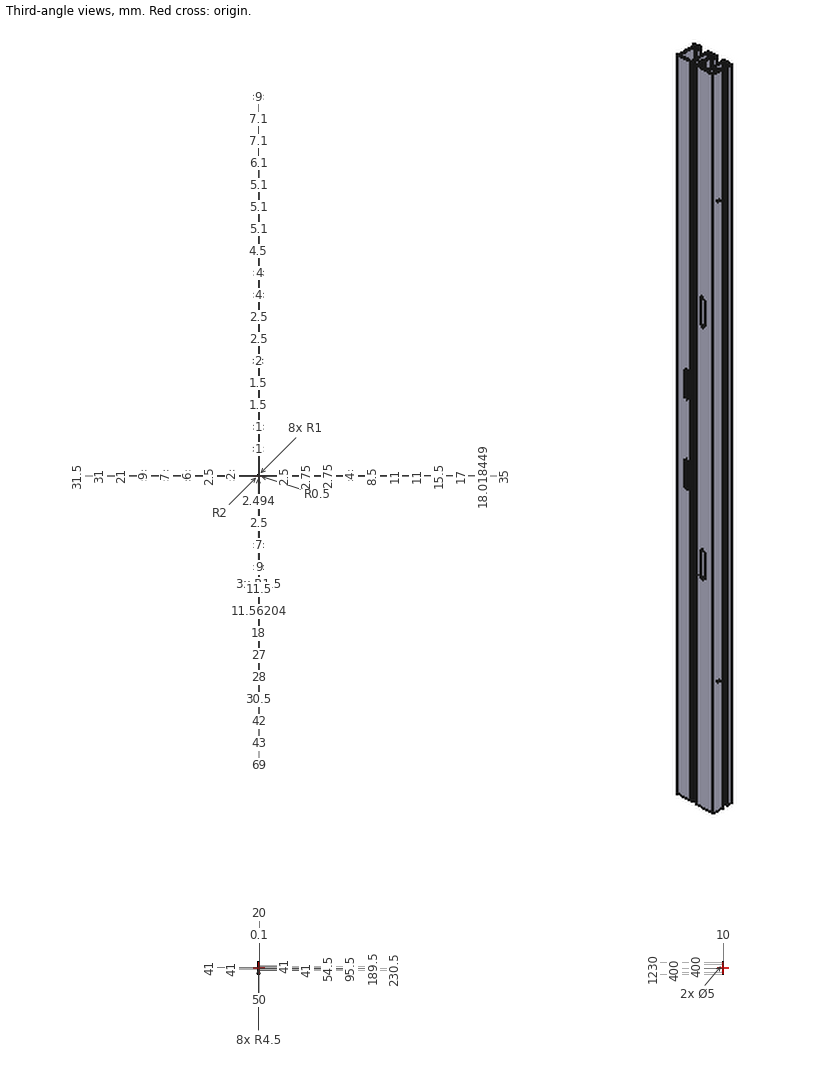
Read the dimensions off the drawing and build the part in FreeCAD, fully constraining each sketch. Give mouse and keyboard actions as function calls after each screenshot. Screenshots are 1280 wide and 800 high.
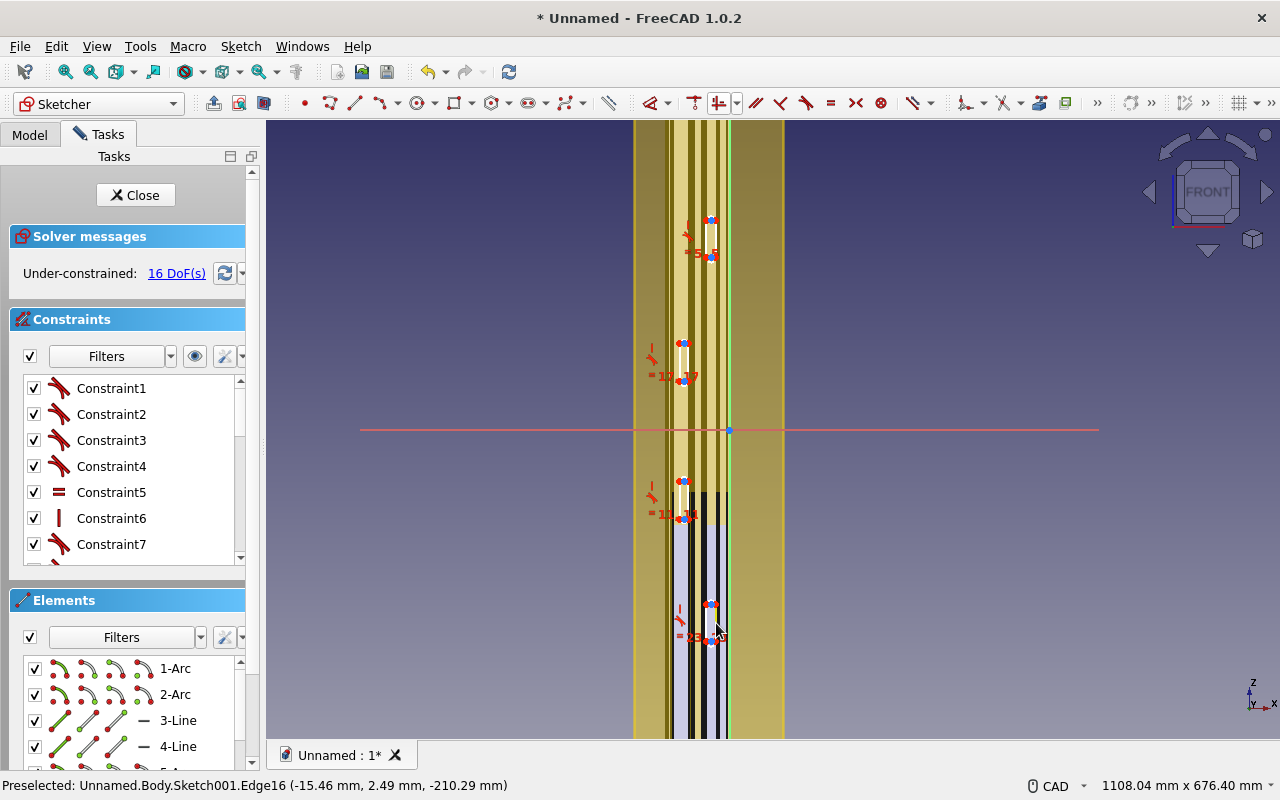
scroll(708, 262, up, 6)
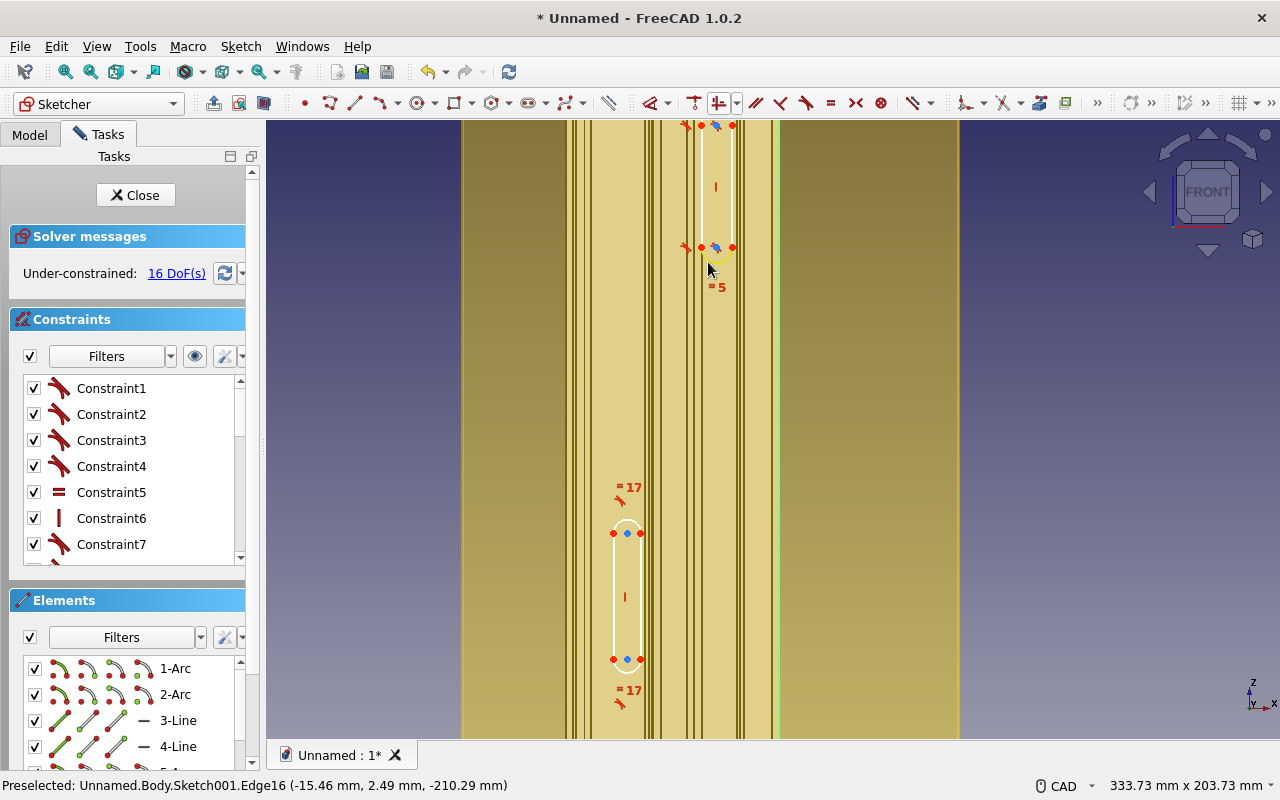
click(708, 260)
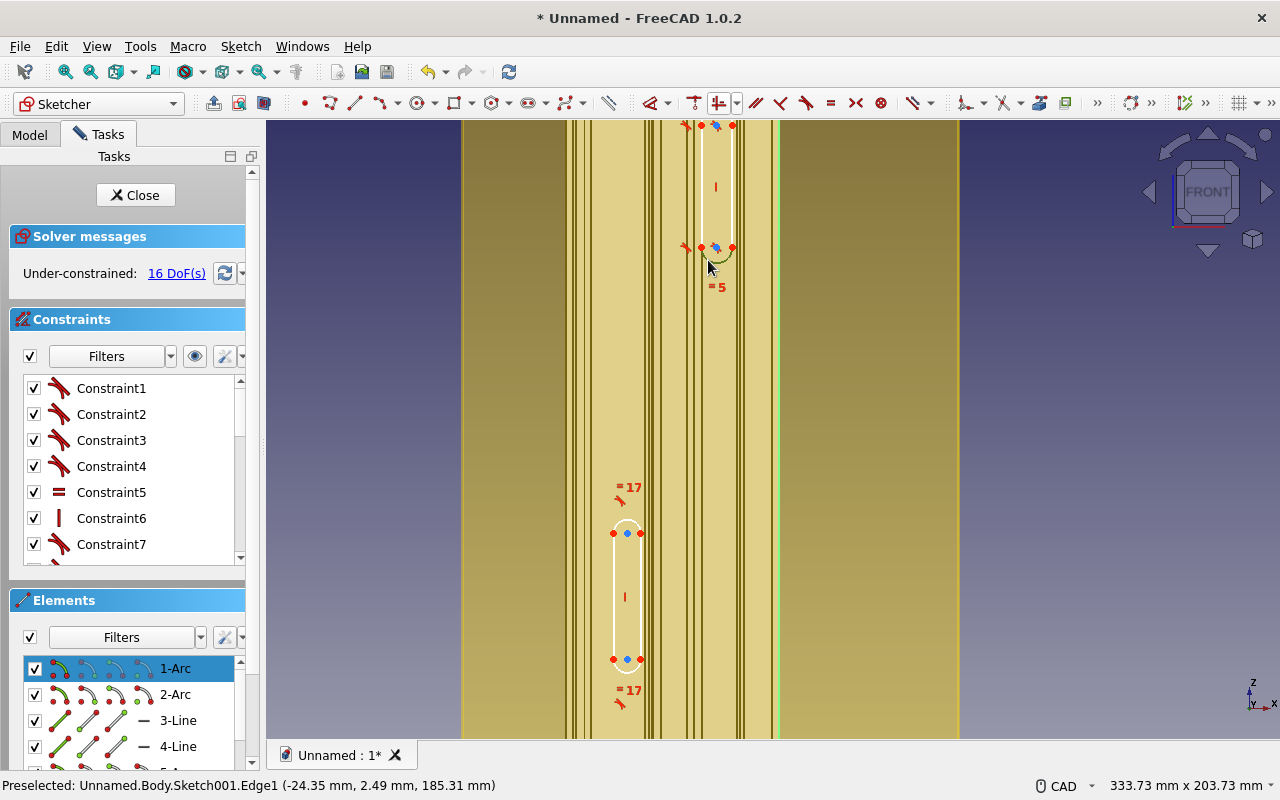
scroll(708, 261, down, 6)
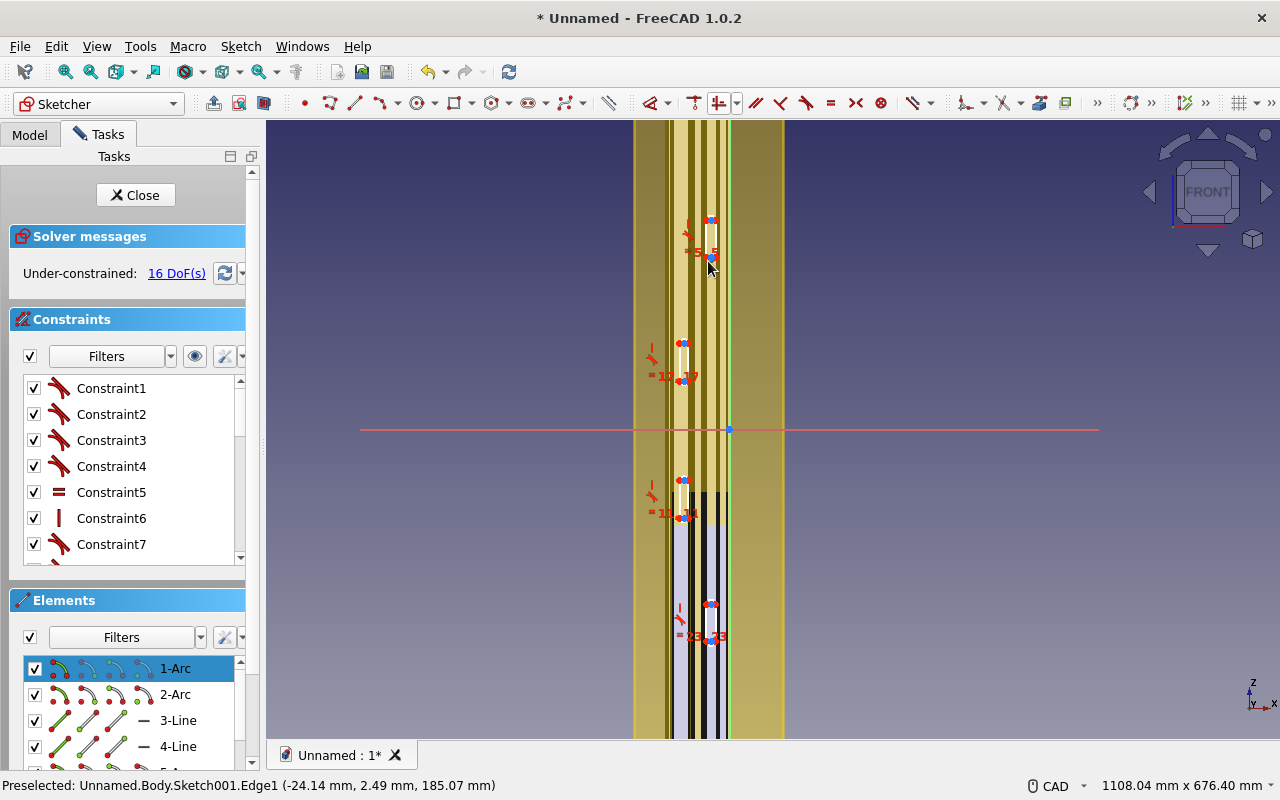
scroll(682, 522, up, 7)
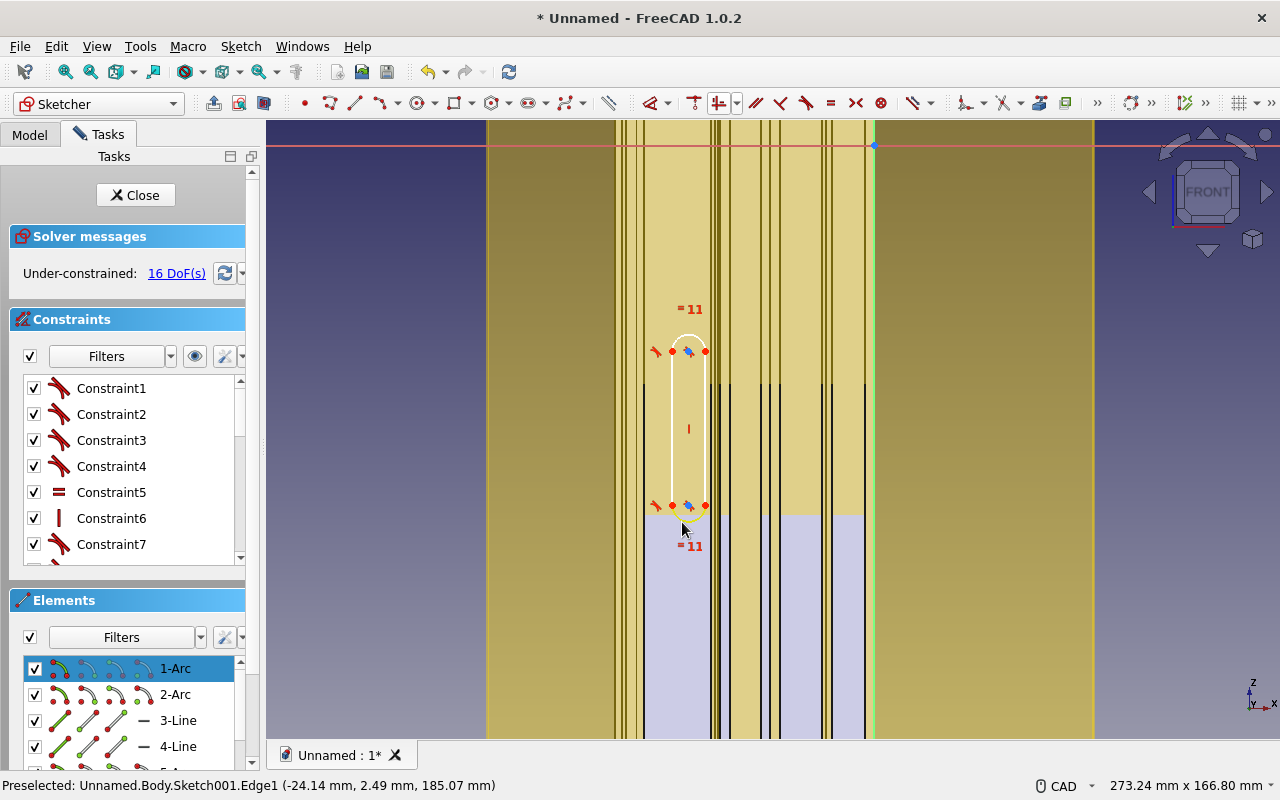
click(679, 519)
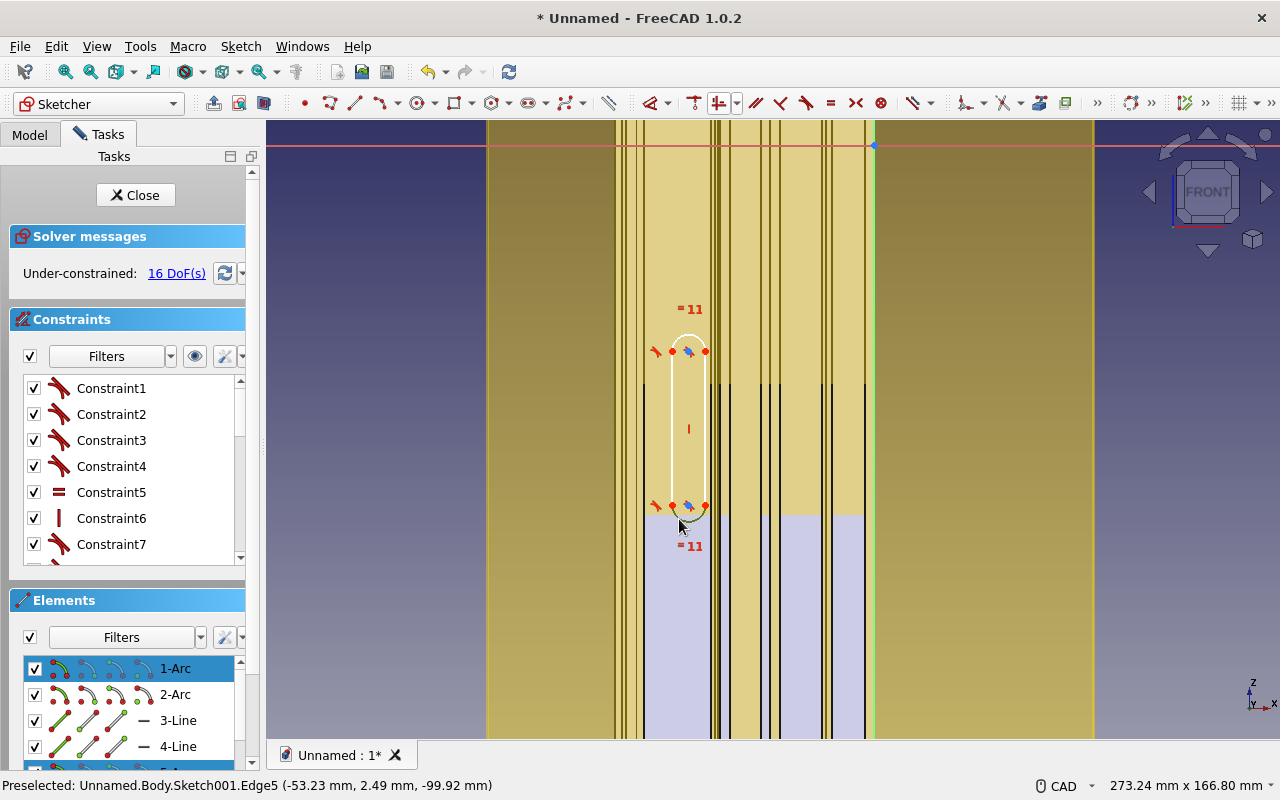
scroll(682, 522, down, 7)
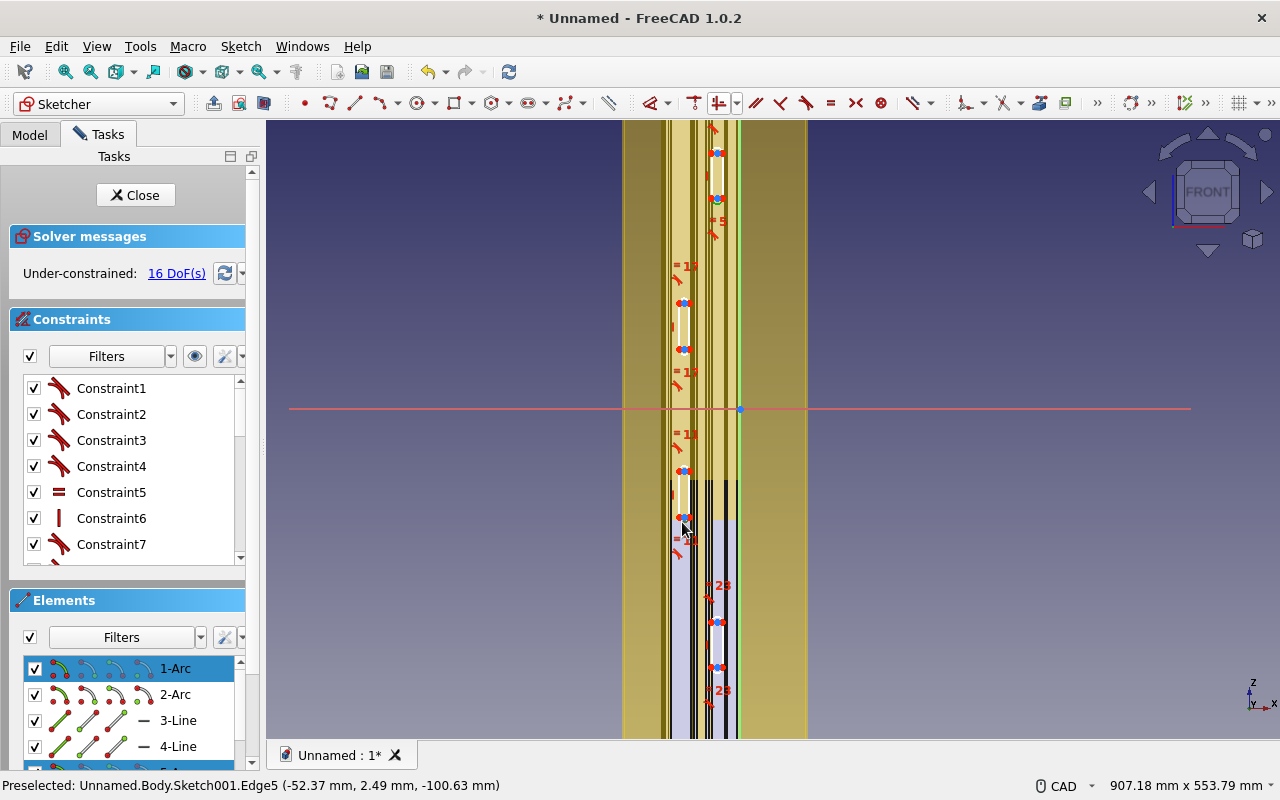
scroll(682, 384, up, 7)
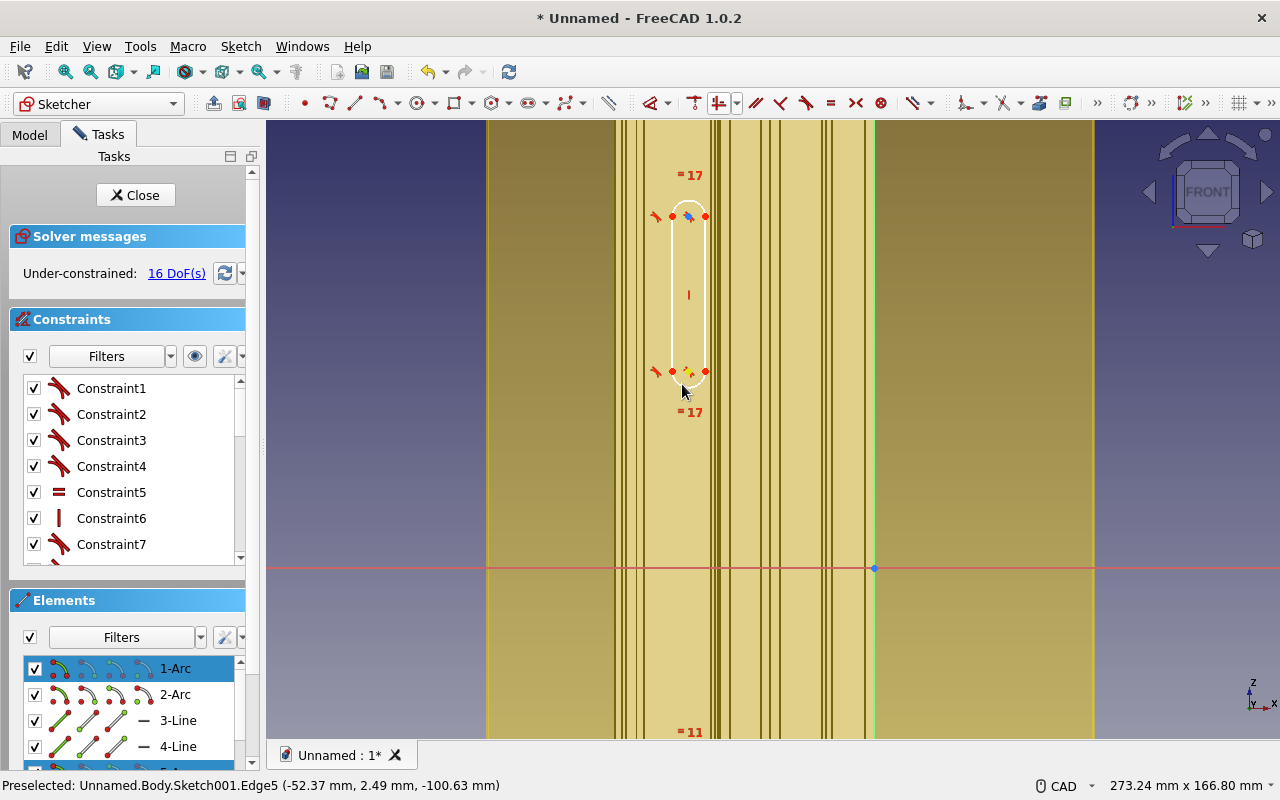
click(679, 384)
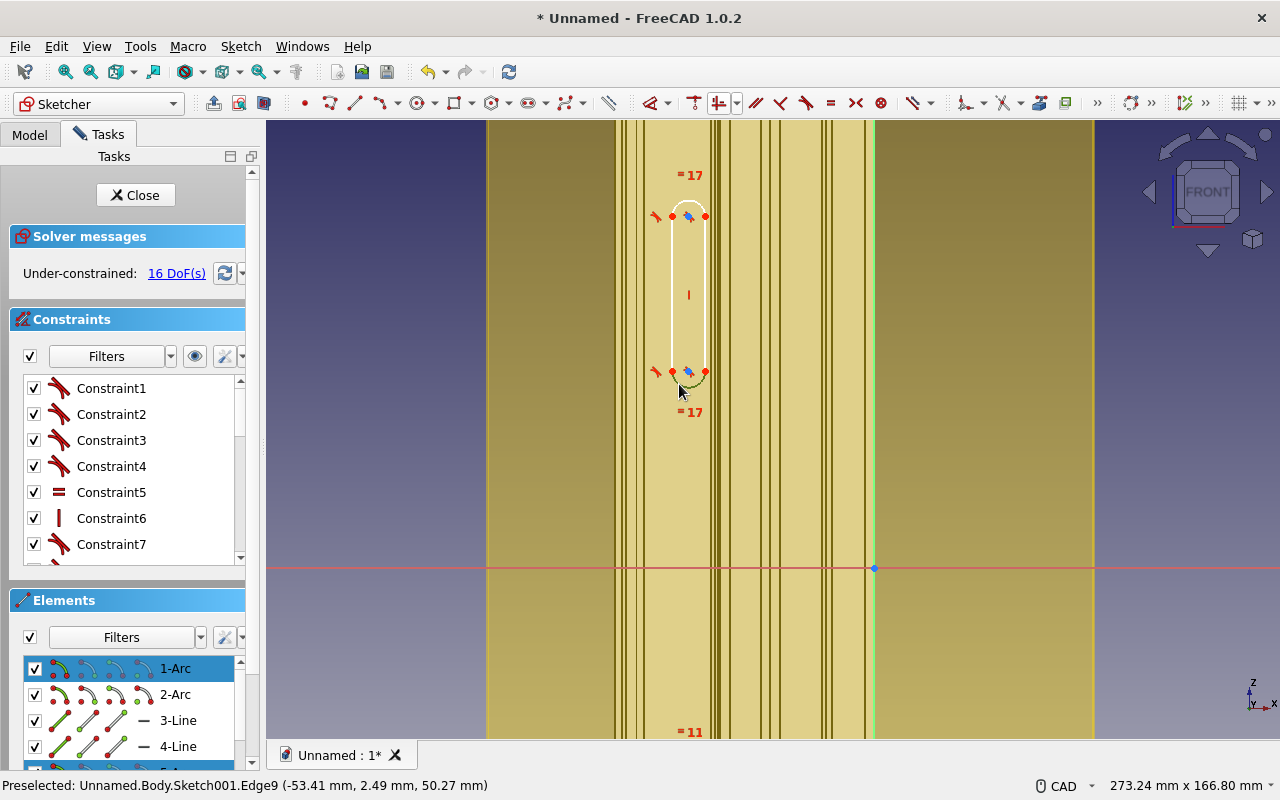
scroll(682, 384, down, 7)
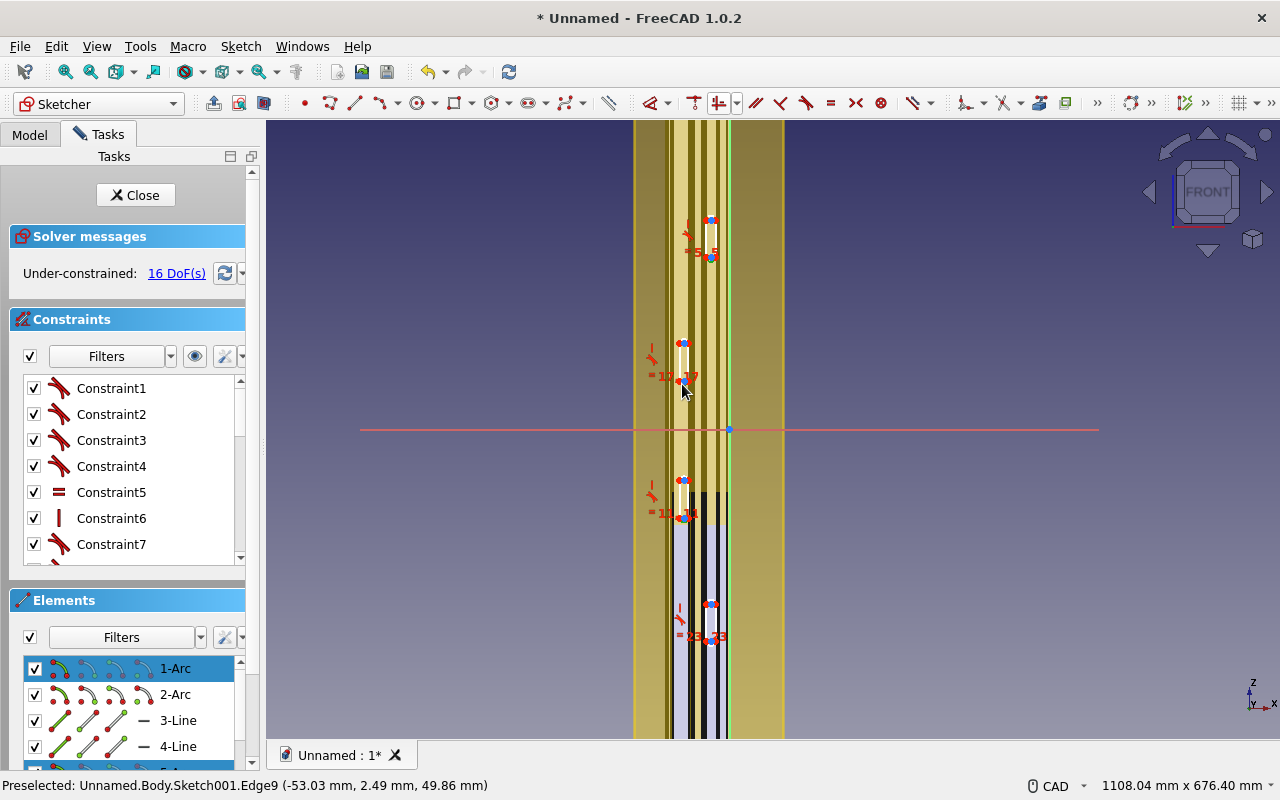
scroll(708, 645, up, 6)